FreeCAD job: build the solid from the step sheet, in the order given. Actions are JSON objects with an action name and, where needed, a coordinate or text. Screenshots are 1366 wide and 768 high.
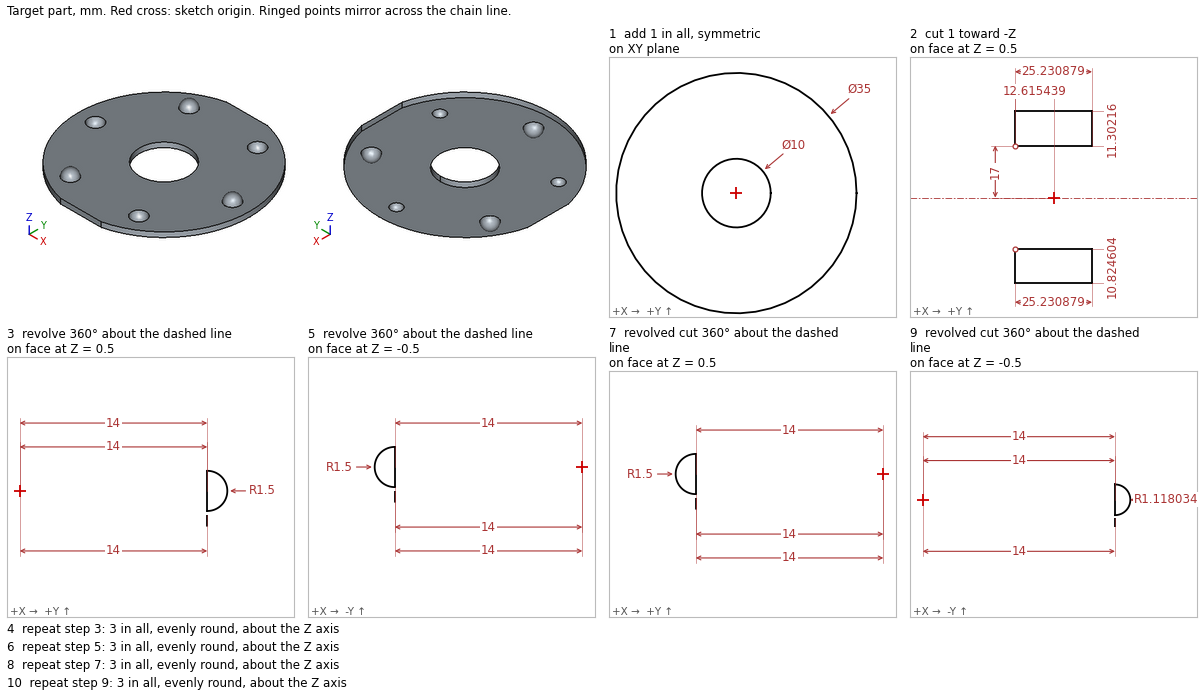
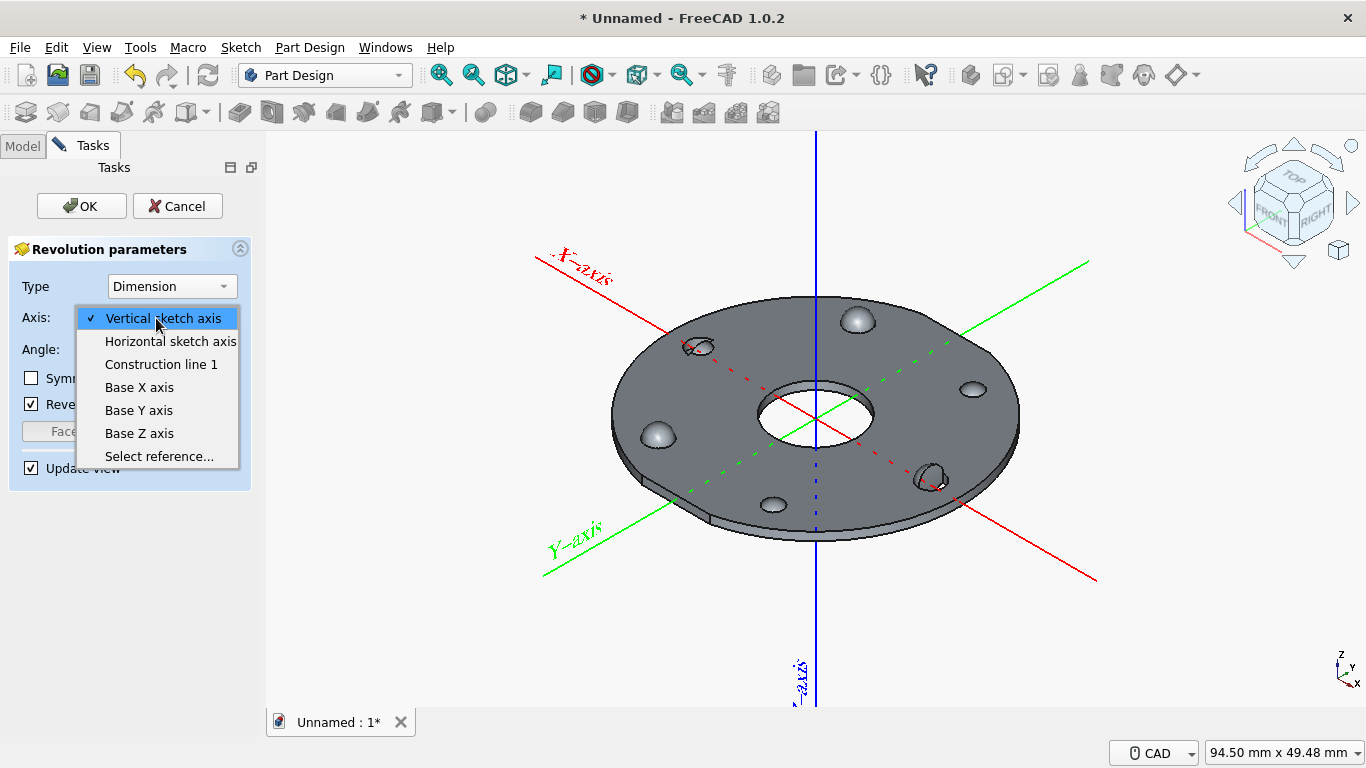
{"action": "left_click", "coordinate": [156, 364]}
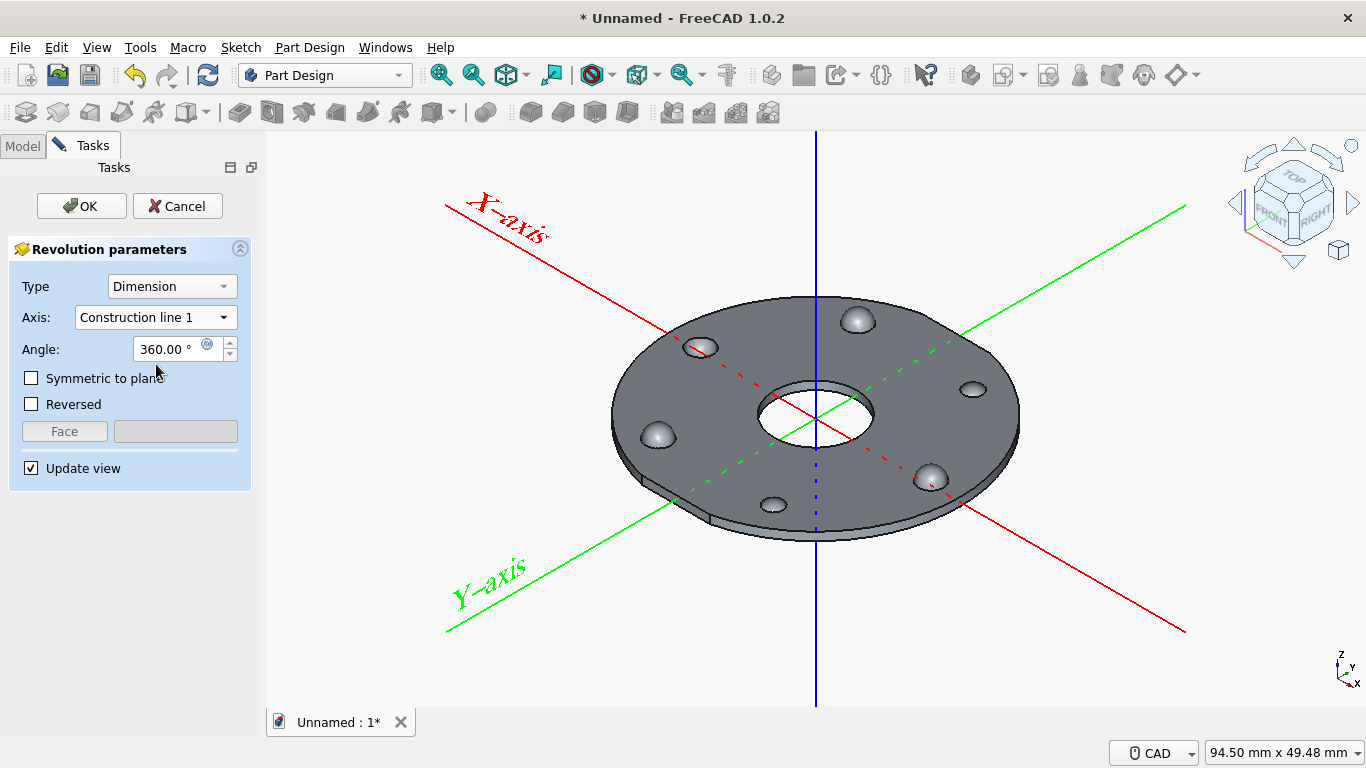
{"action": "left_click", "coordinate": [82, 206]}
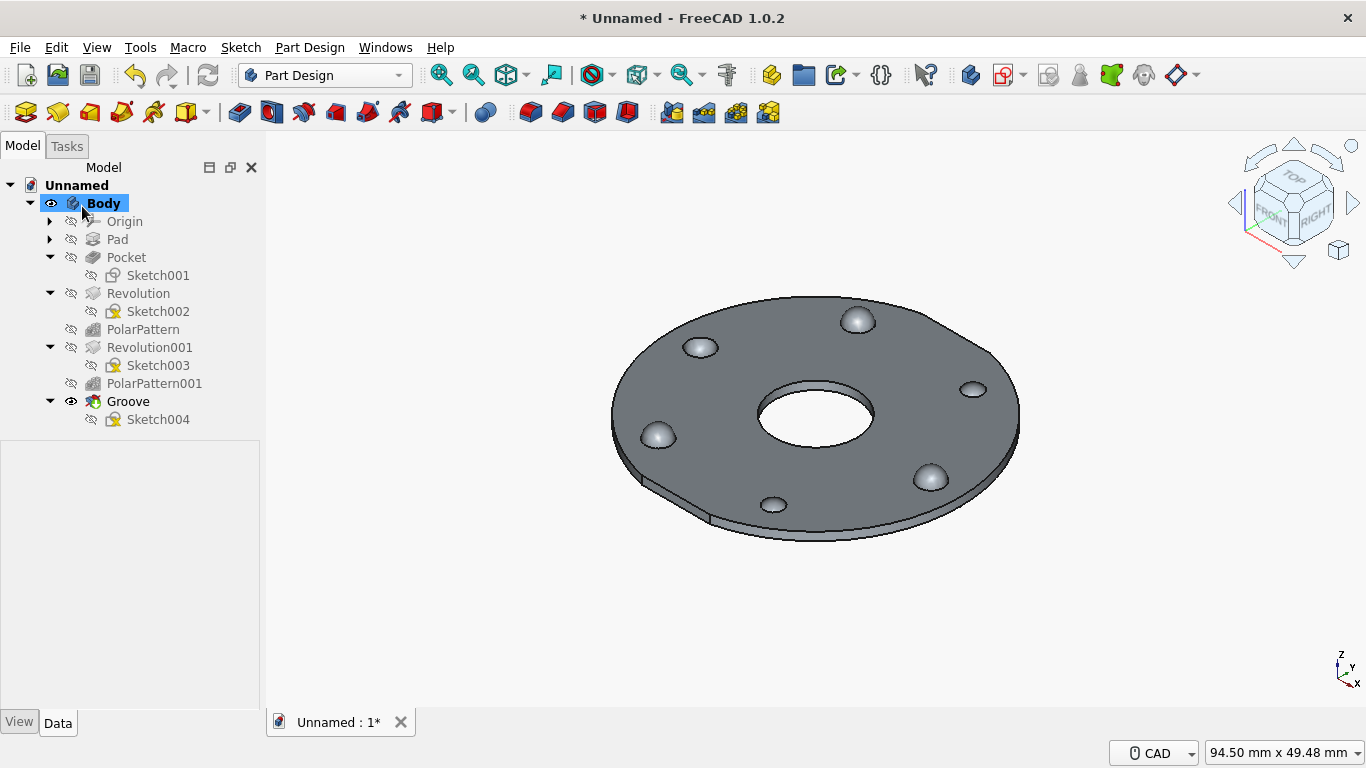
{"action": "left_click", "coordinate": [116, 401]}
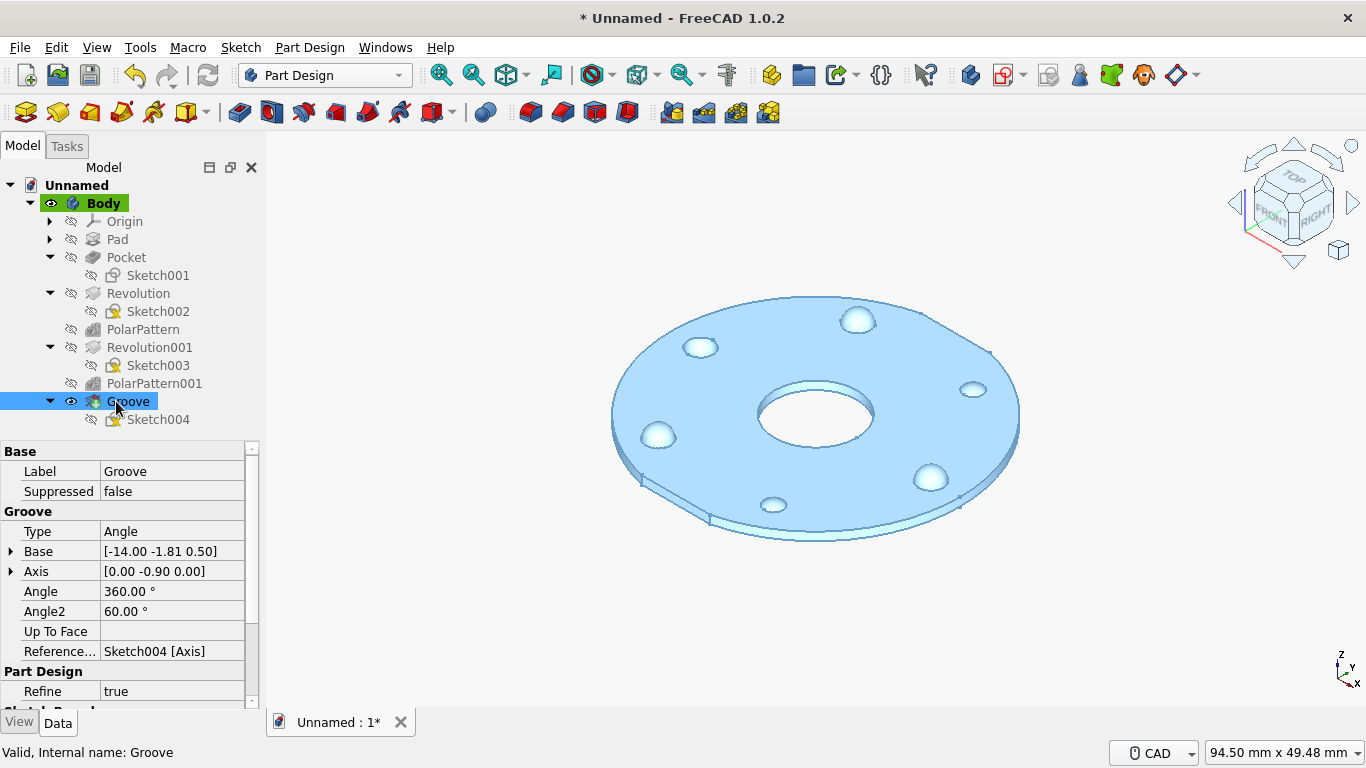
{"action": "left_click", "coordinate": [736, 112]}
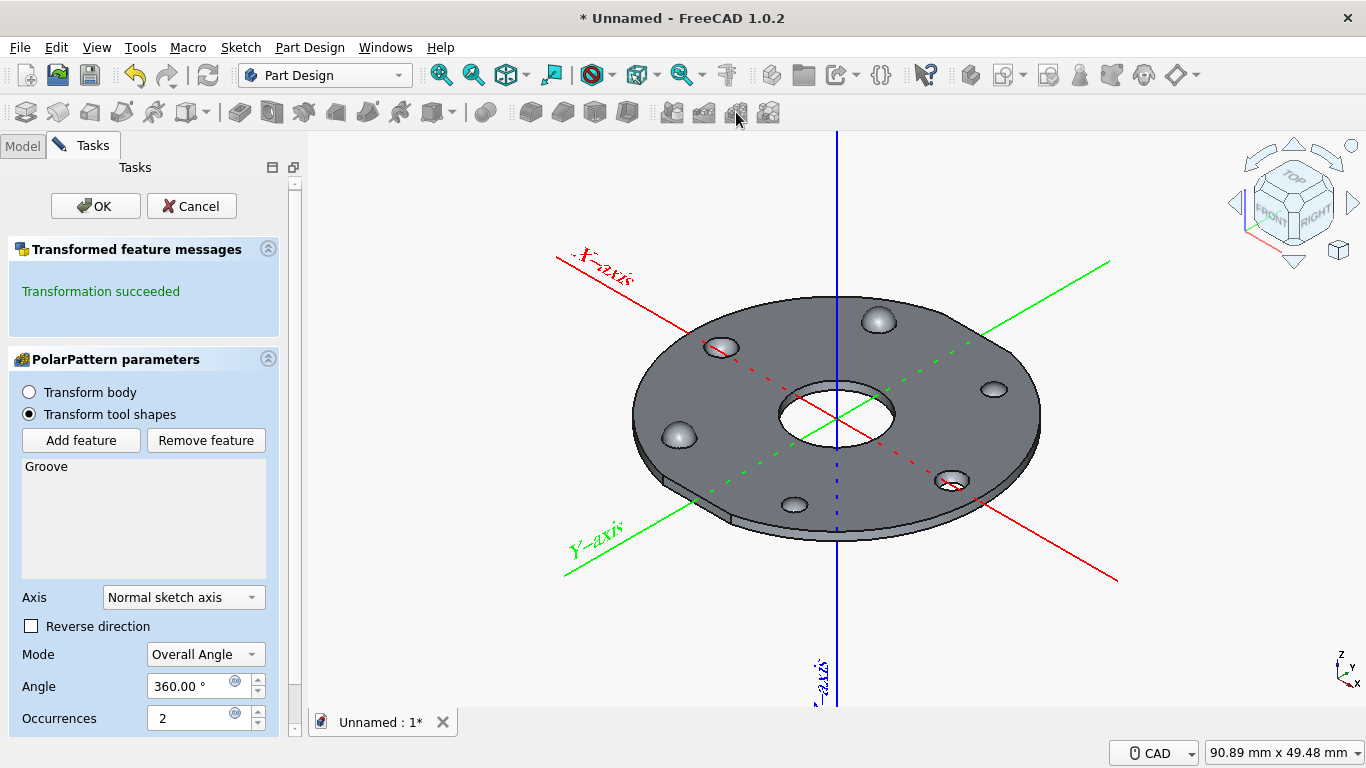
{"action": "left_click", "coordinate": [184, 598]}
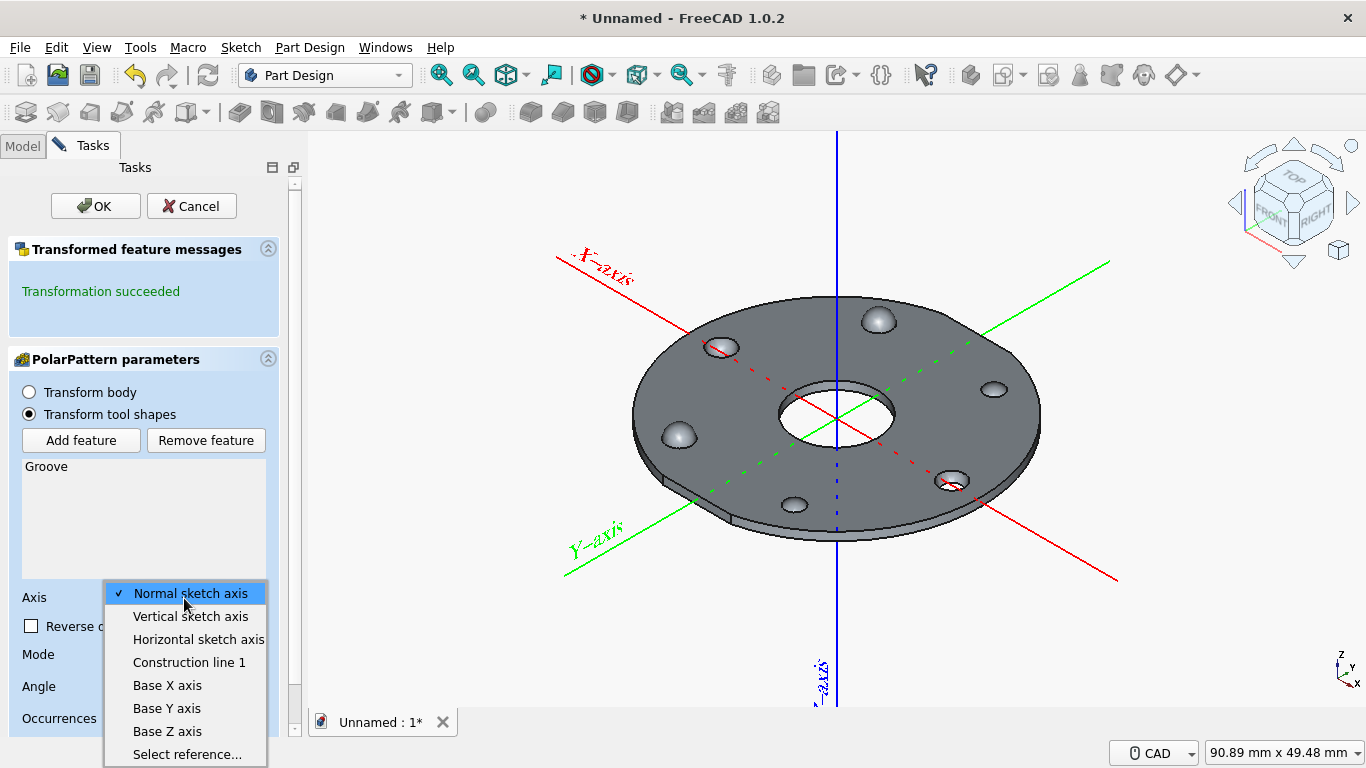
{"action": "left_click", "coordinate": [184, 732]}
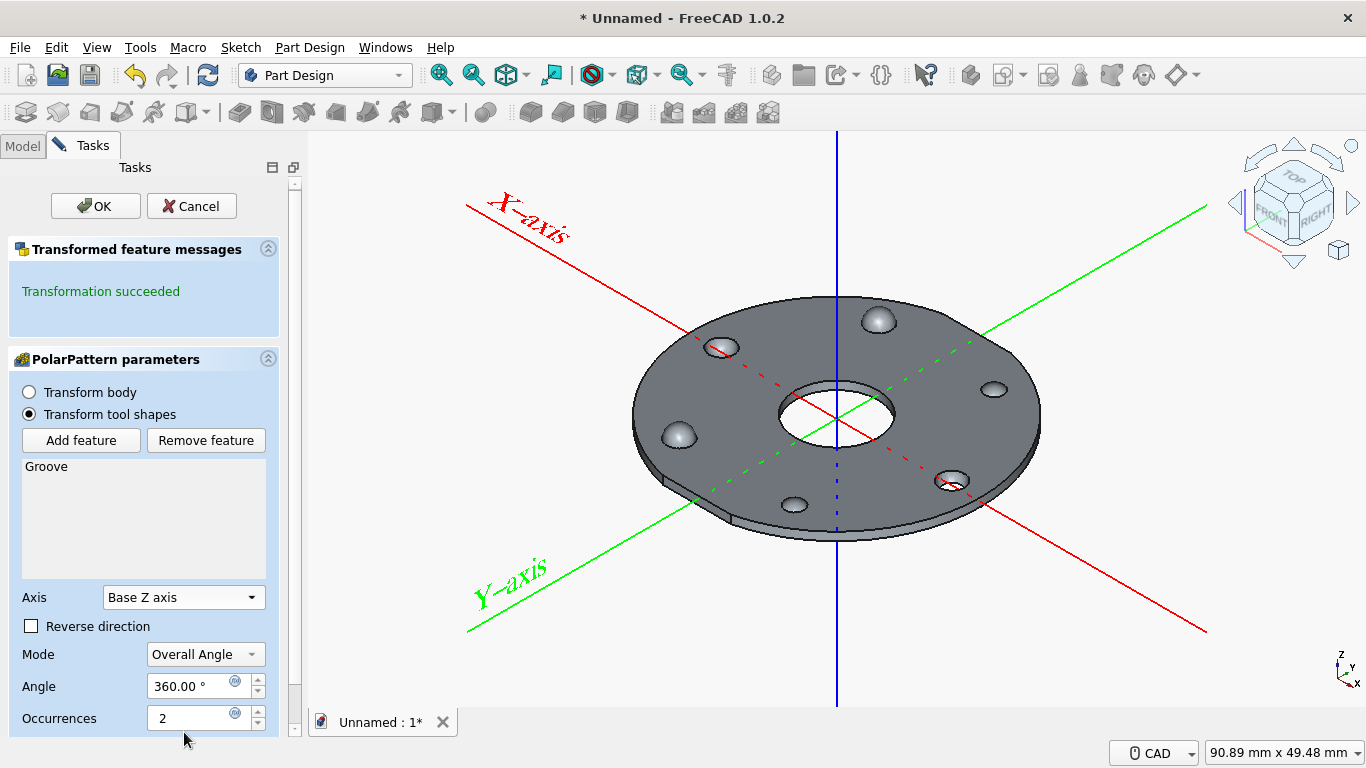
{"action": "triple_click", "coordinate": [198, 718]}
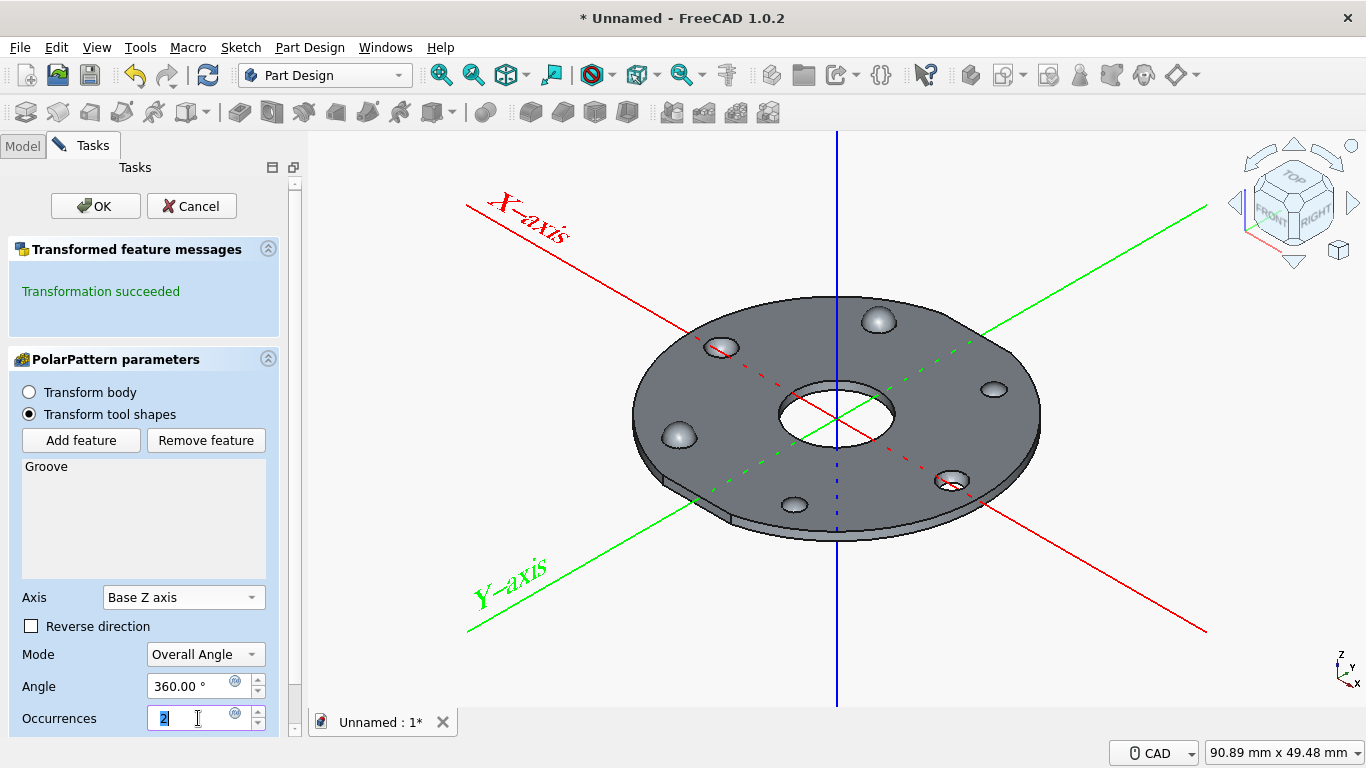
{"action": "type", "text": "3"}
{"action": "key", "text": "Tab"}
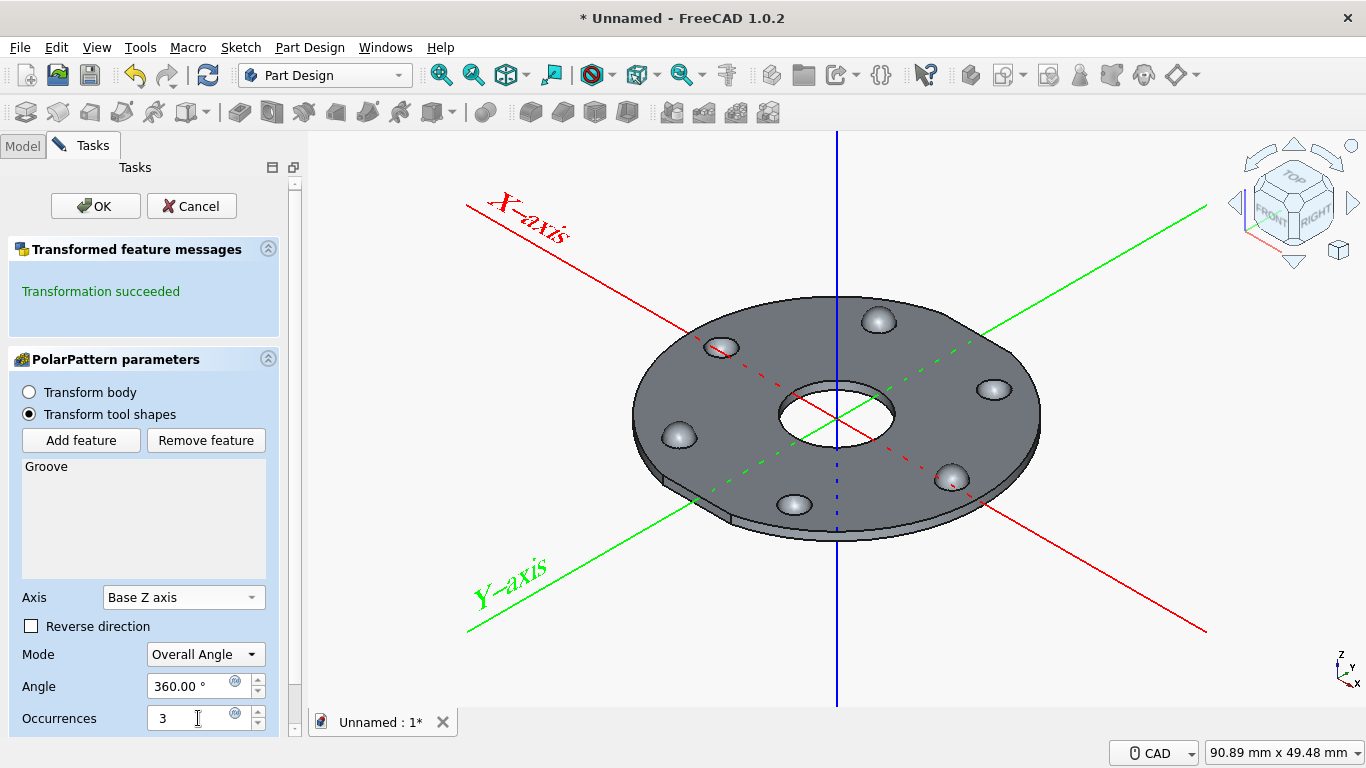
{"action": "left_click", "coordinate": [96, 206]}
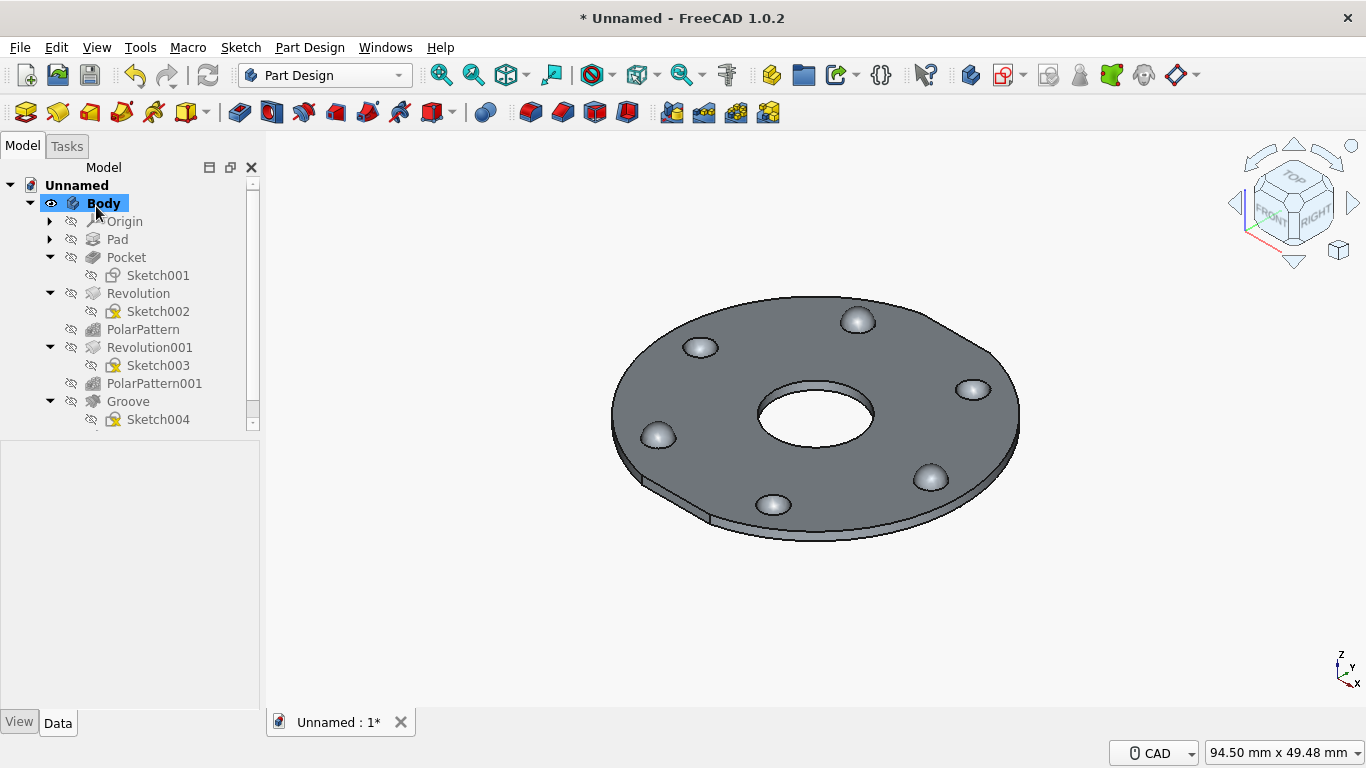
{"action": "key", "text": "5"}